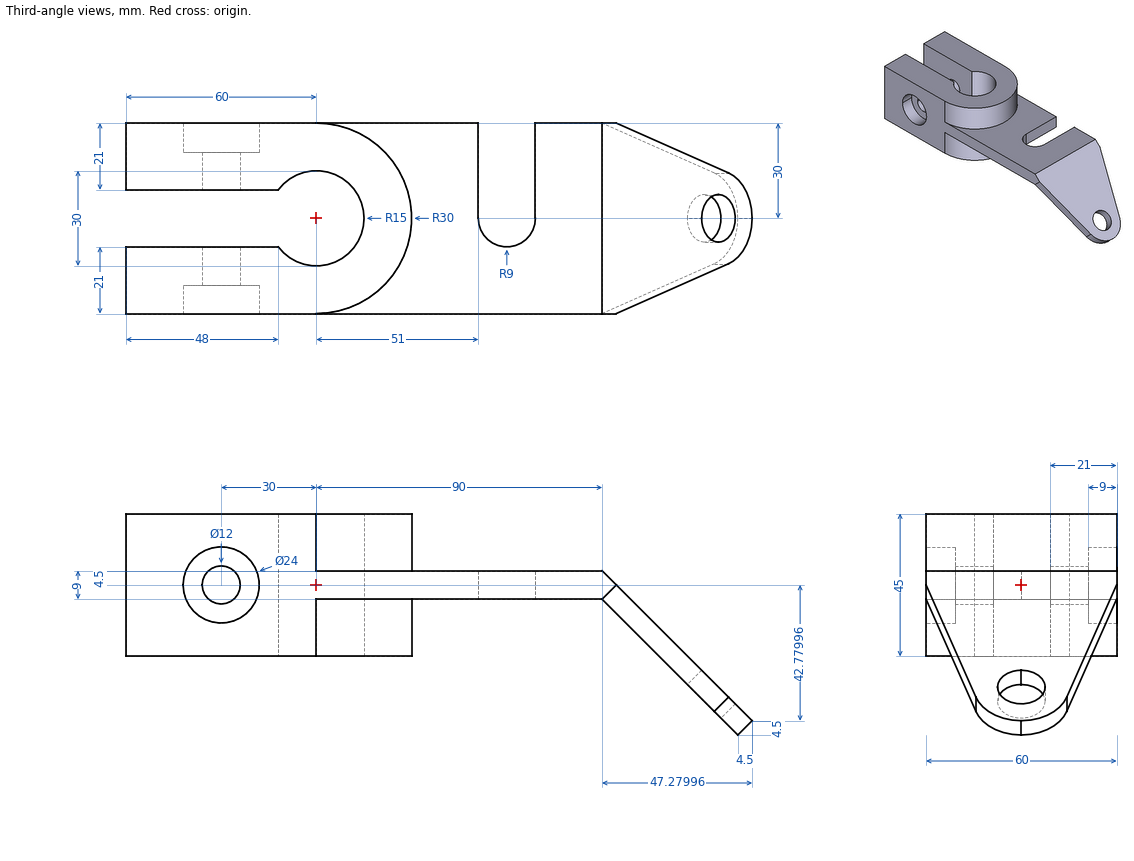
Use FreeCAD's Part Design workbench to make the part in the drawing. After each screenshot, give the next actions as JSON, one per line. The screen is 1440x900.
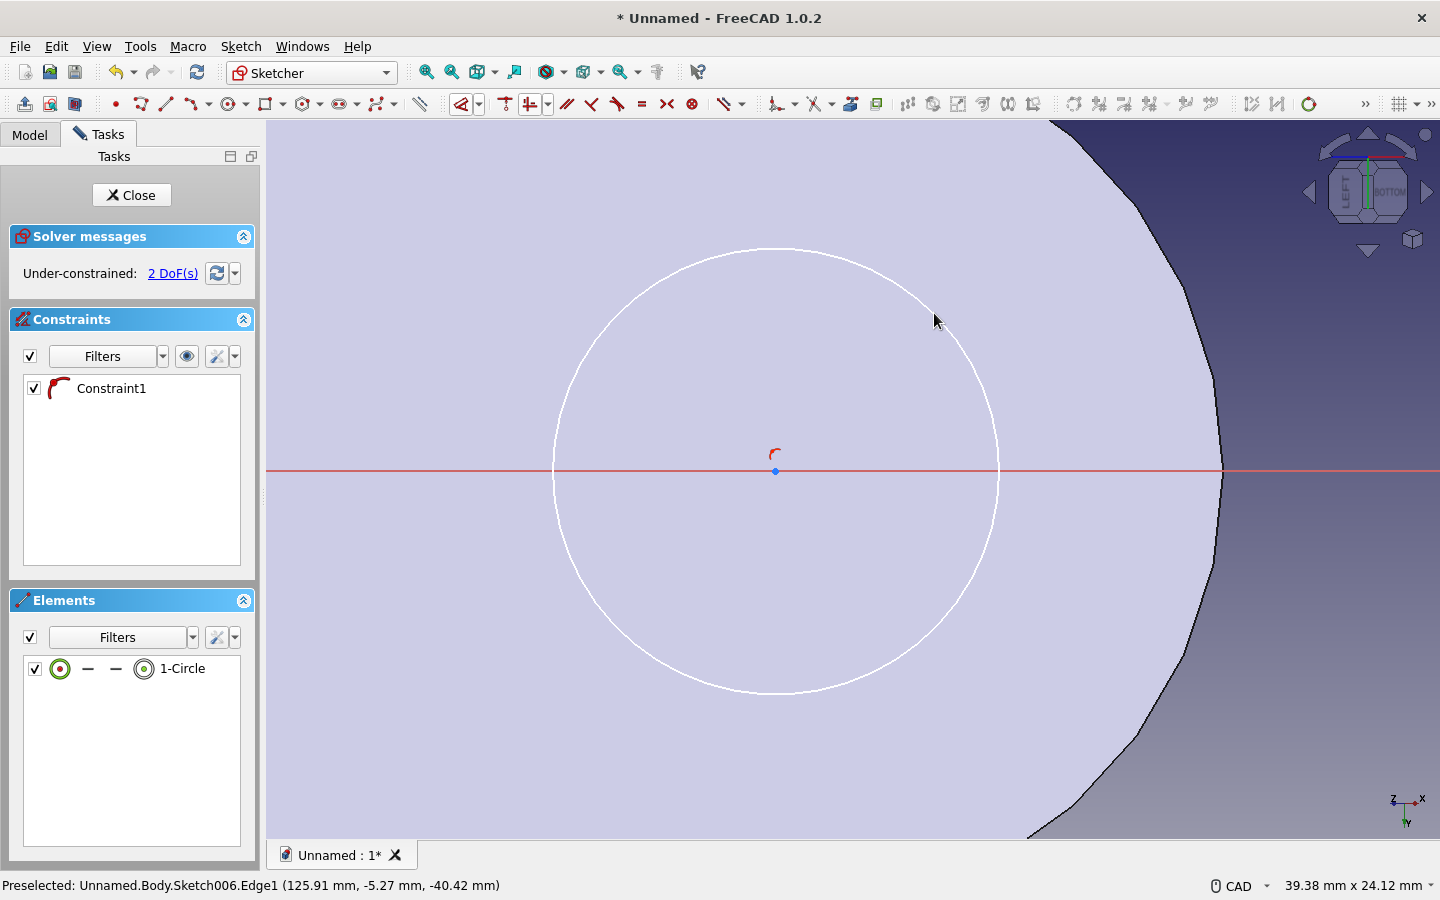
{"action": "left_click", "coordinate": [933, 313]}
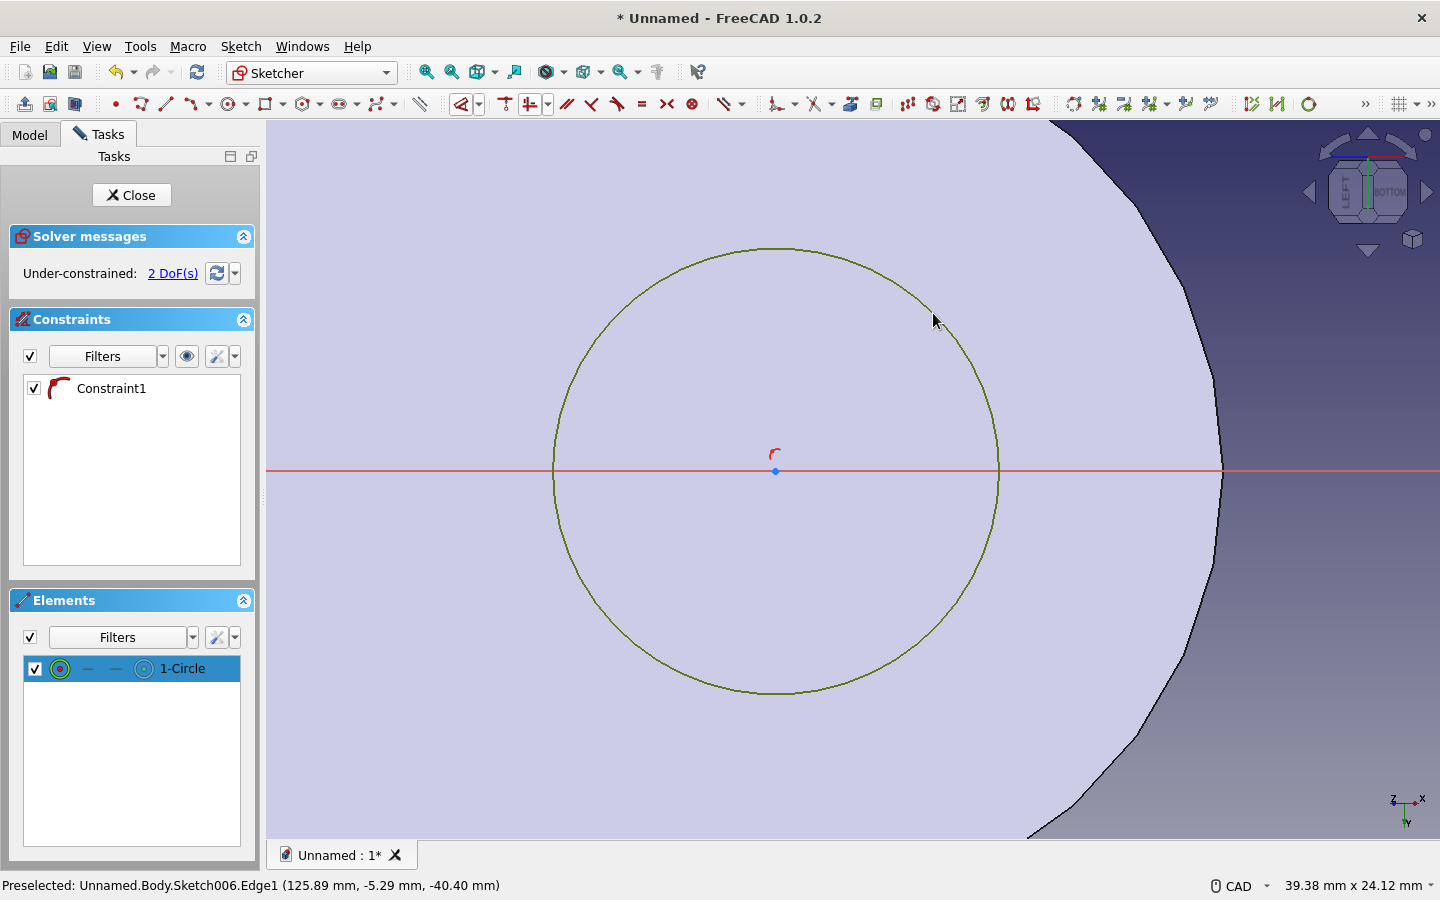
{"action": "left_click", "coordinate": [478, 104]}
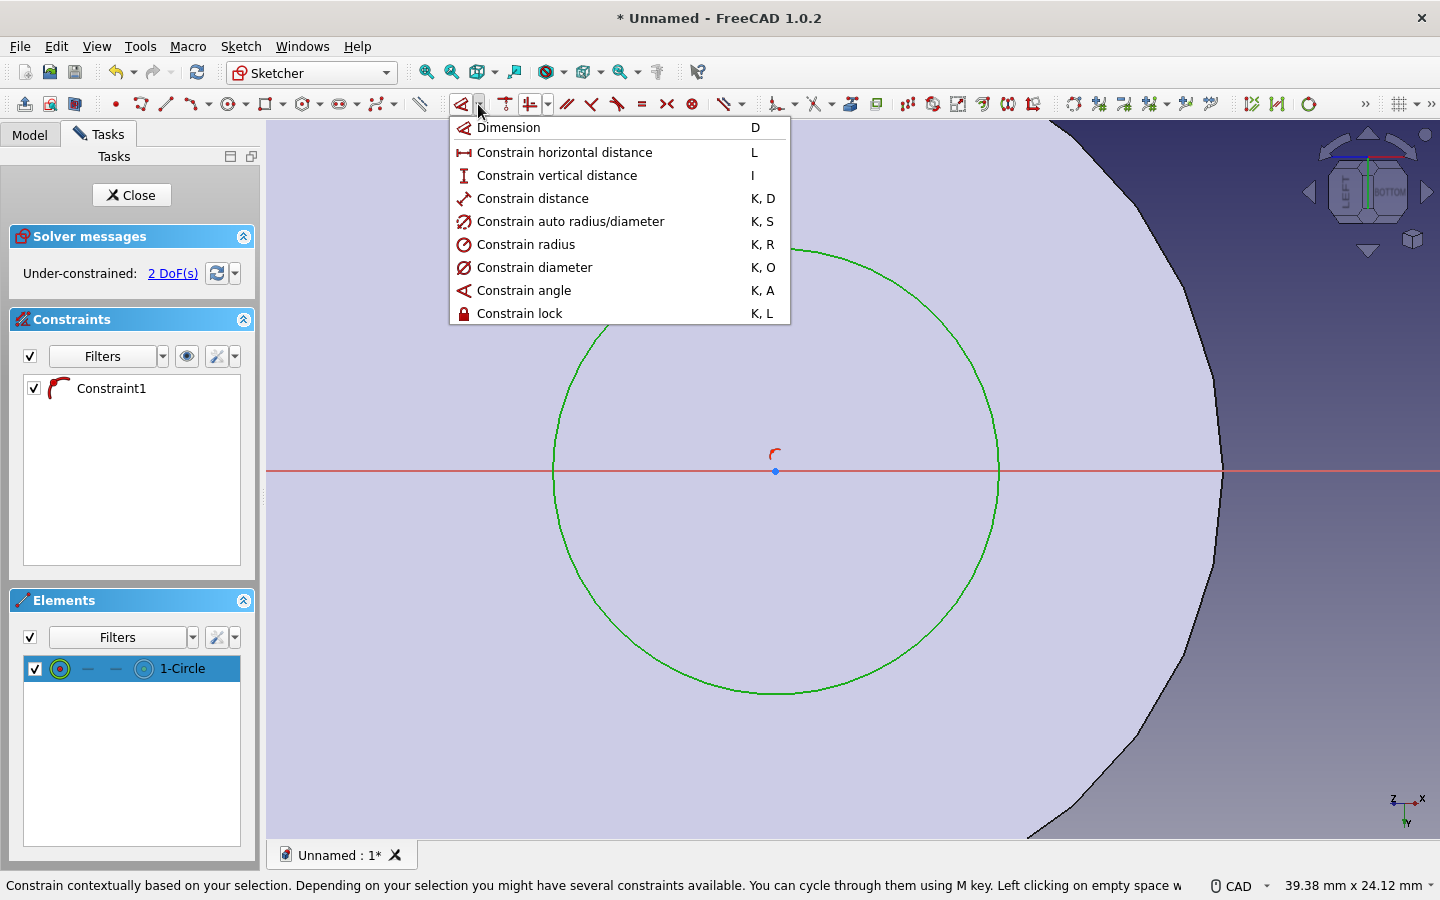
{"action": "left_click", "coordinate": [620, 268]}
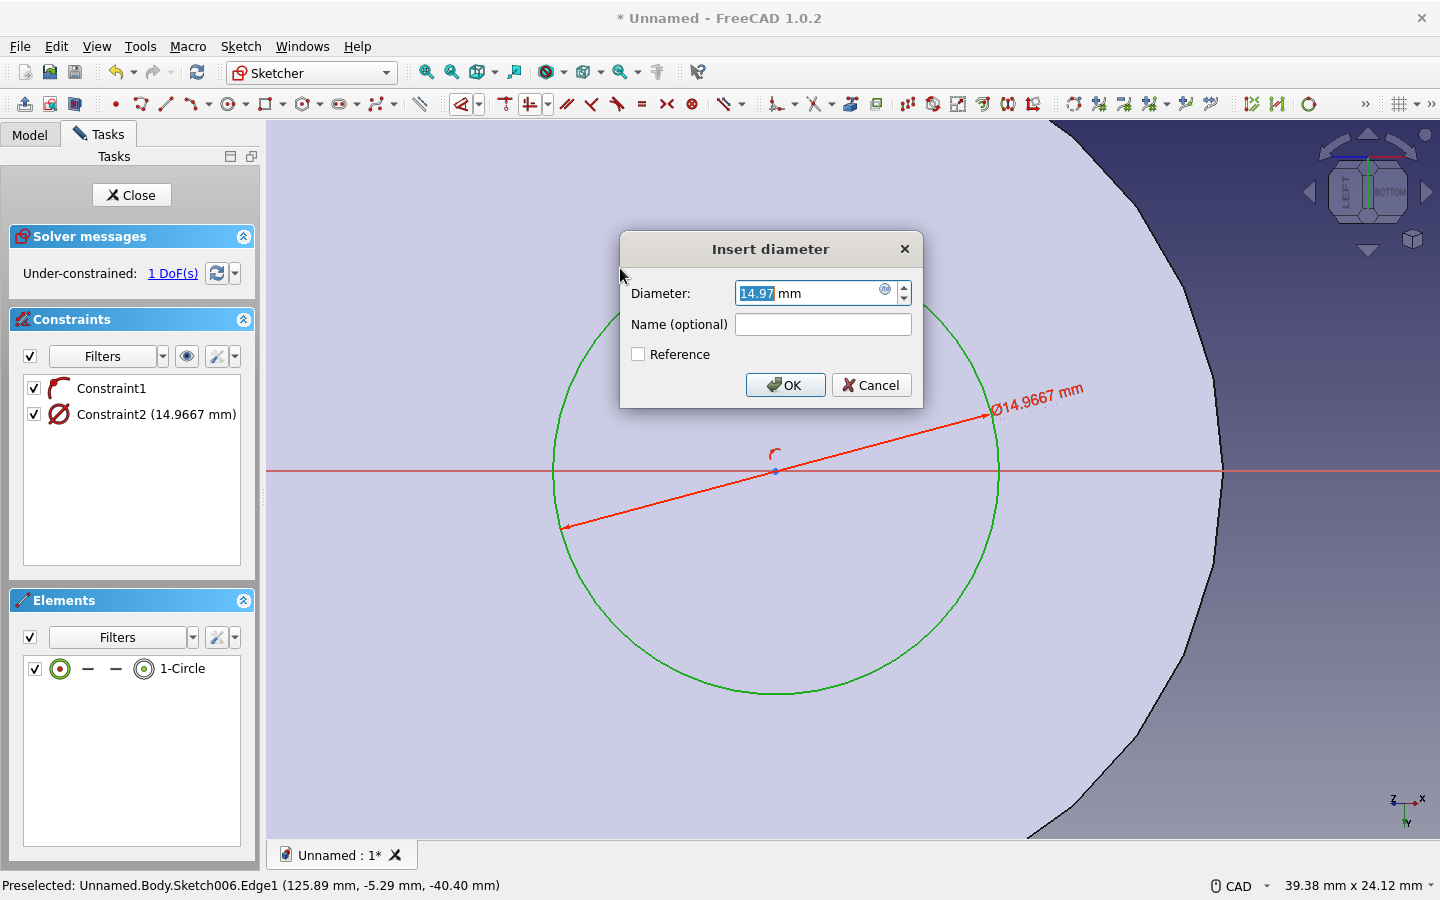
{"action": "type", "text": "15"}
{"action": "key", "text": "Return"}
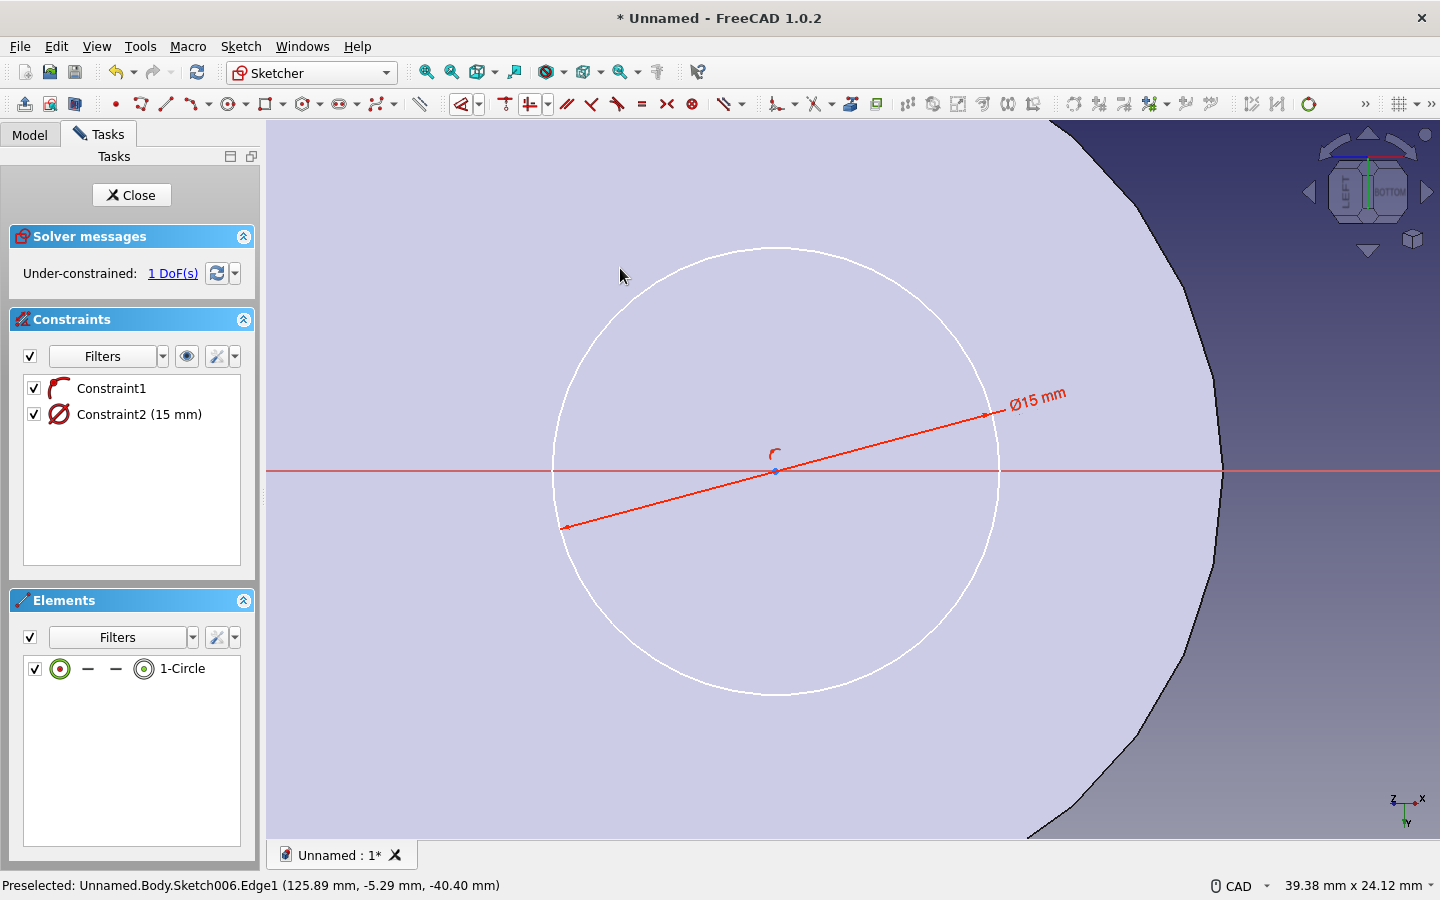
{"action": "left_click", "coordinate": [776, 471]}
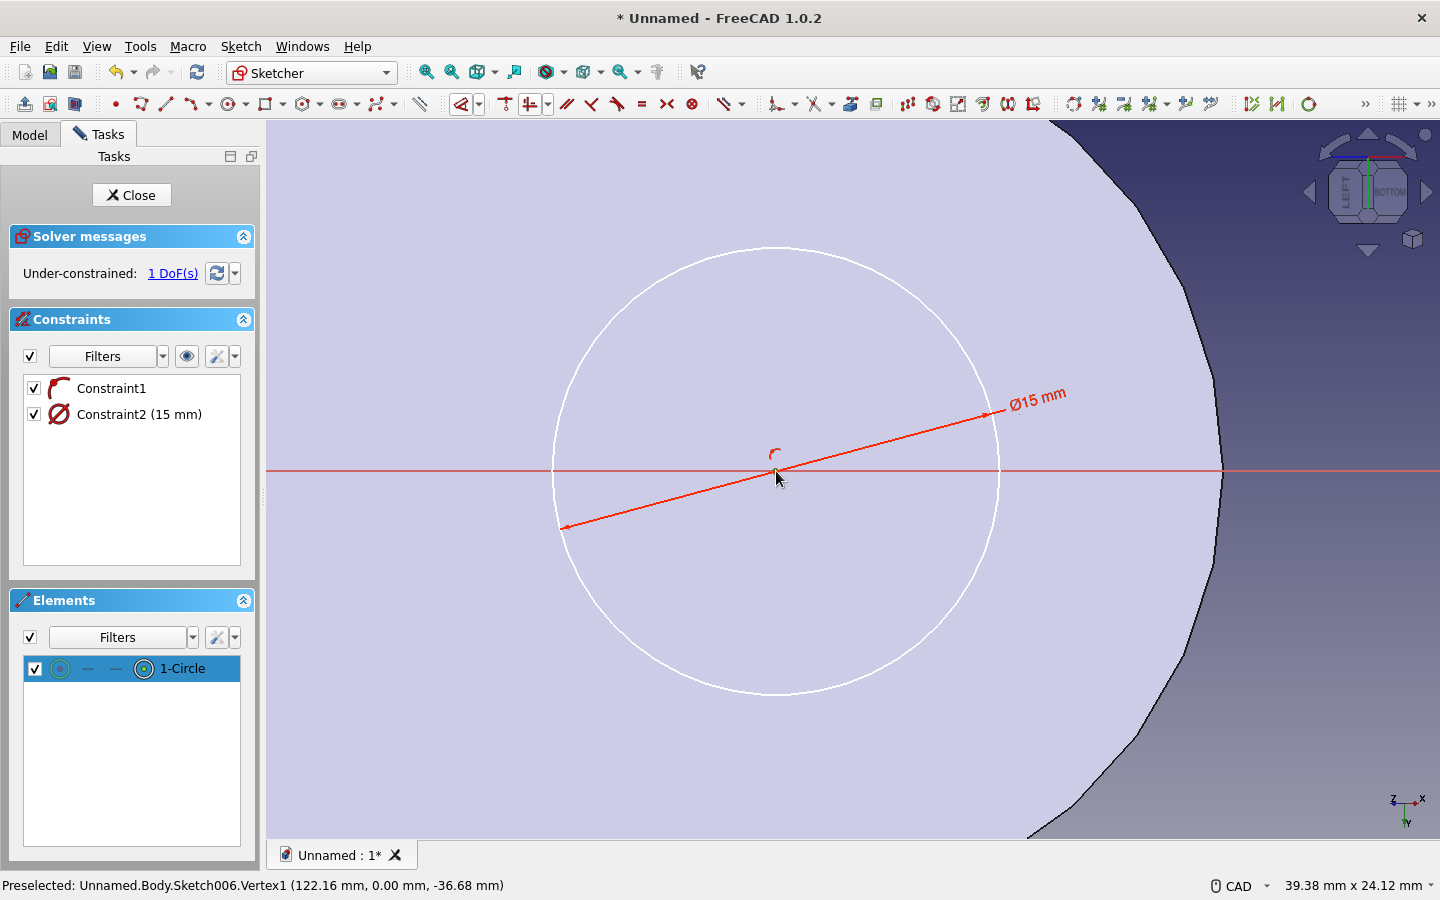
{"action": "key", "text": "l"}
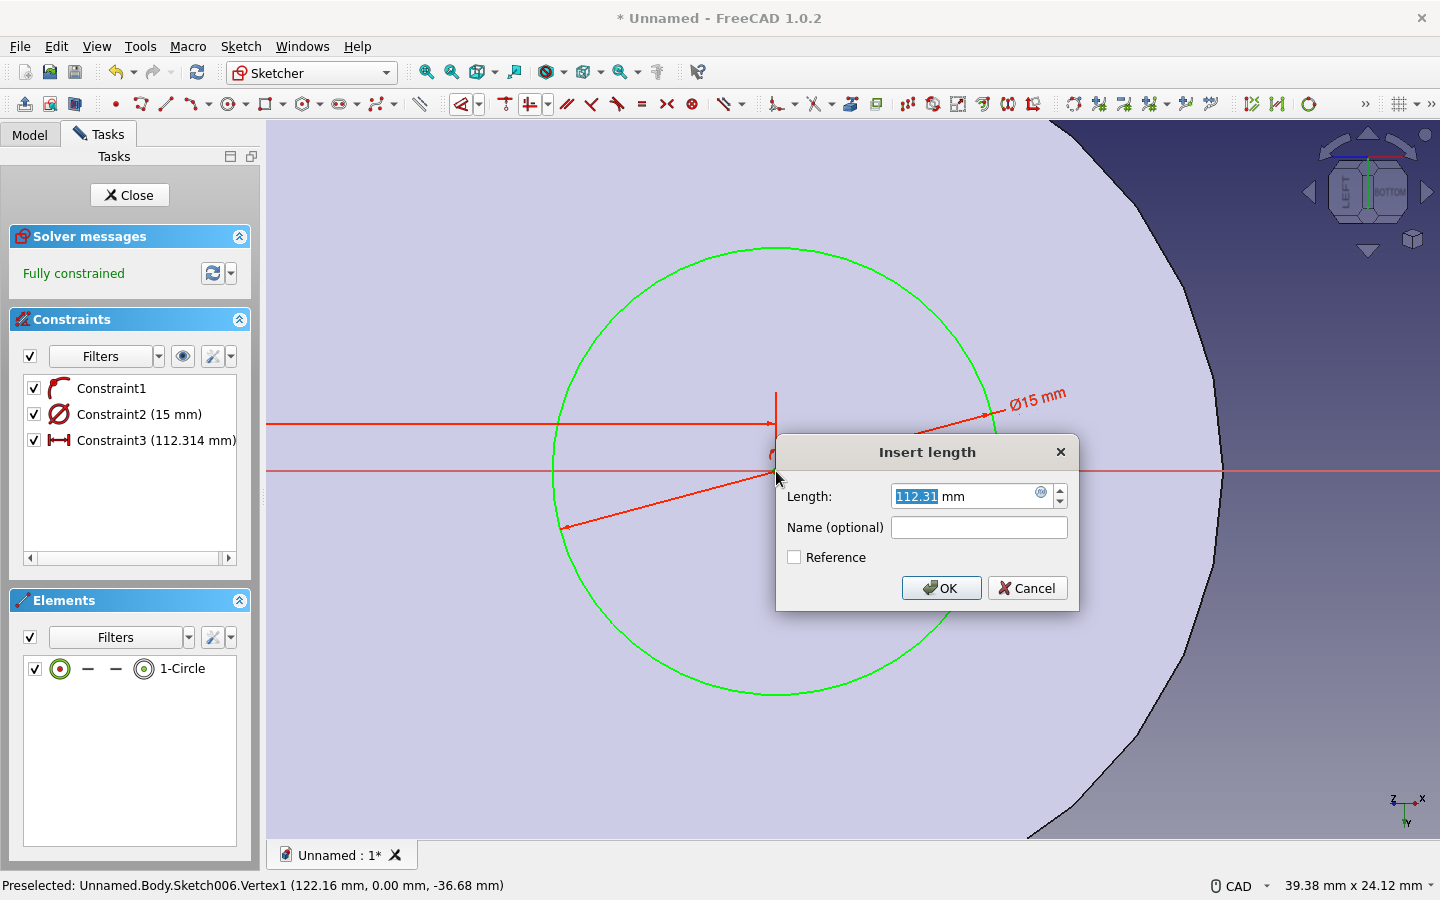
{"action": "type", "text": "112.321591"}
{"action": "key", "text": "Return"}